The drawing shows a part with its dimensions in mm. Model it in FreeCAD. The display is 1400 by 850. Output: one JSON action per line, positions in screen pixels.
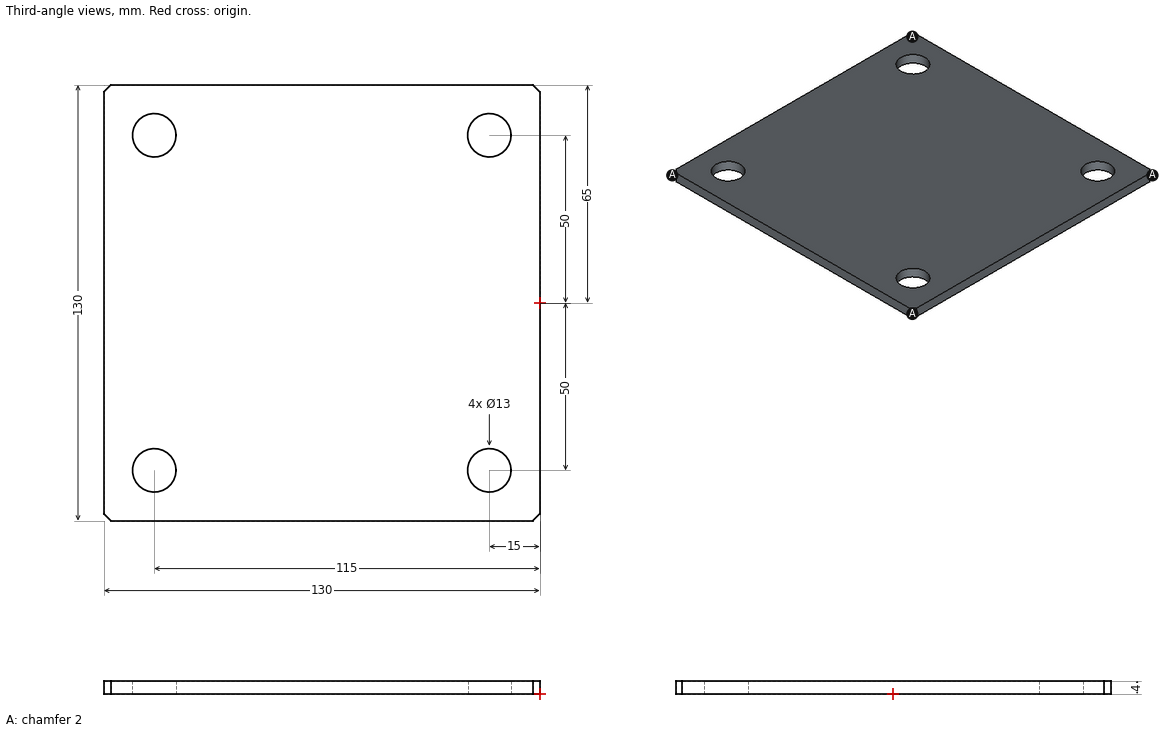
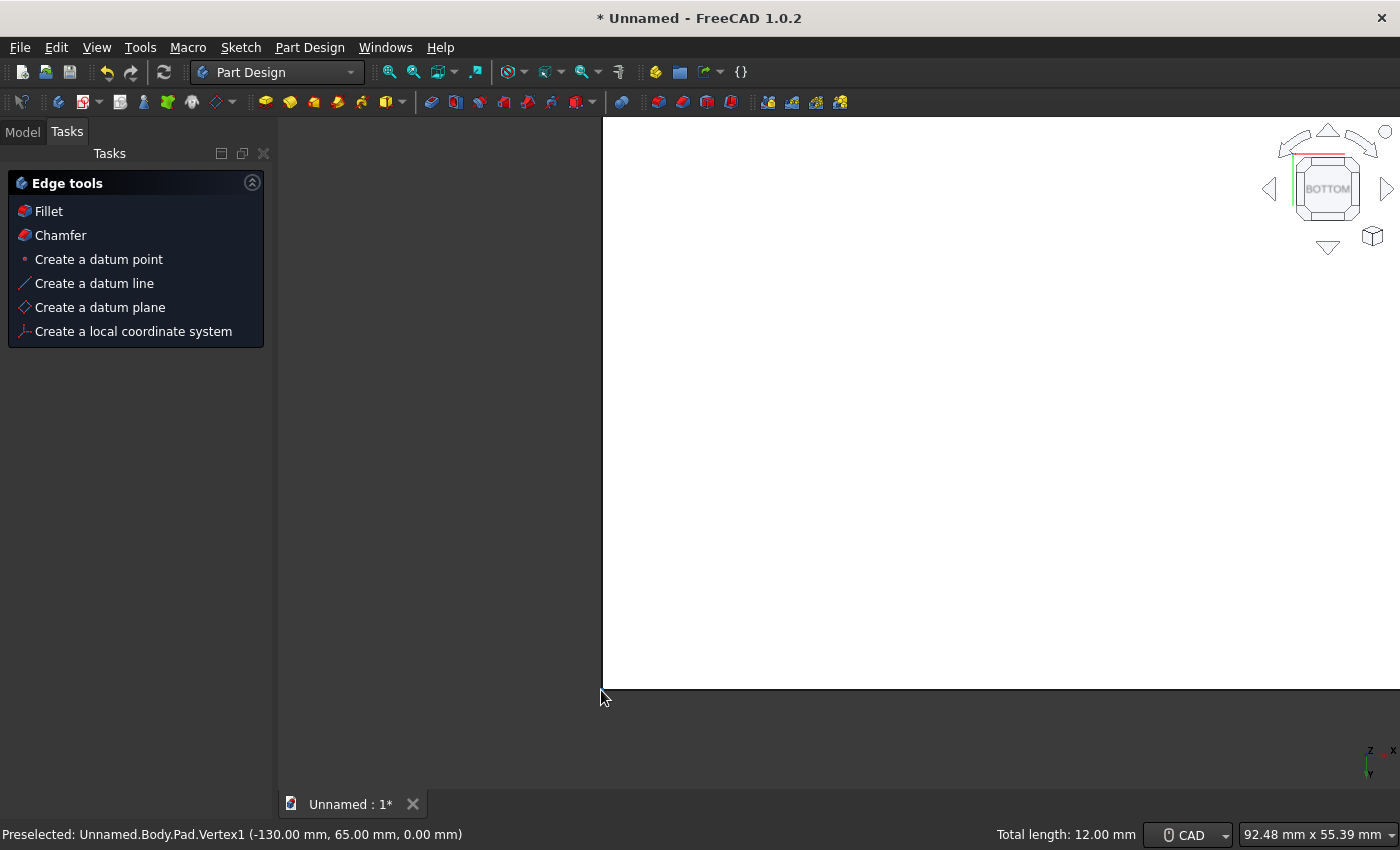
{"action": "left_click", "coordinate": [390, 72]}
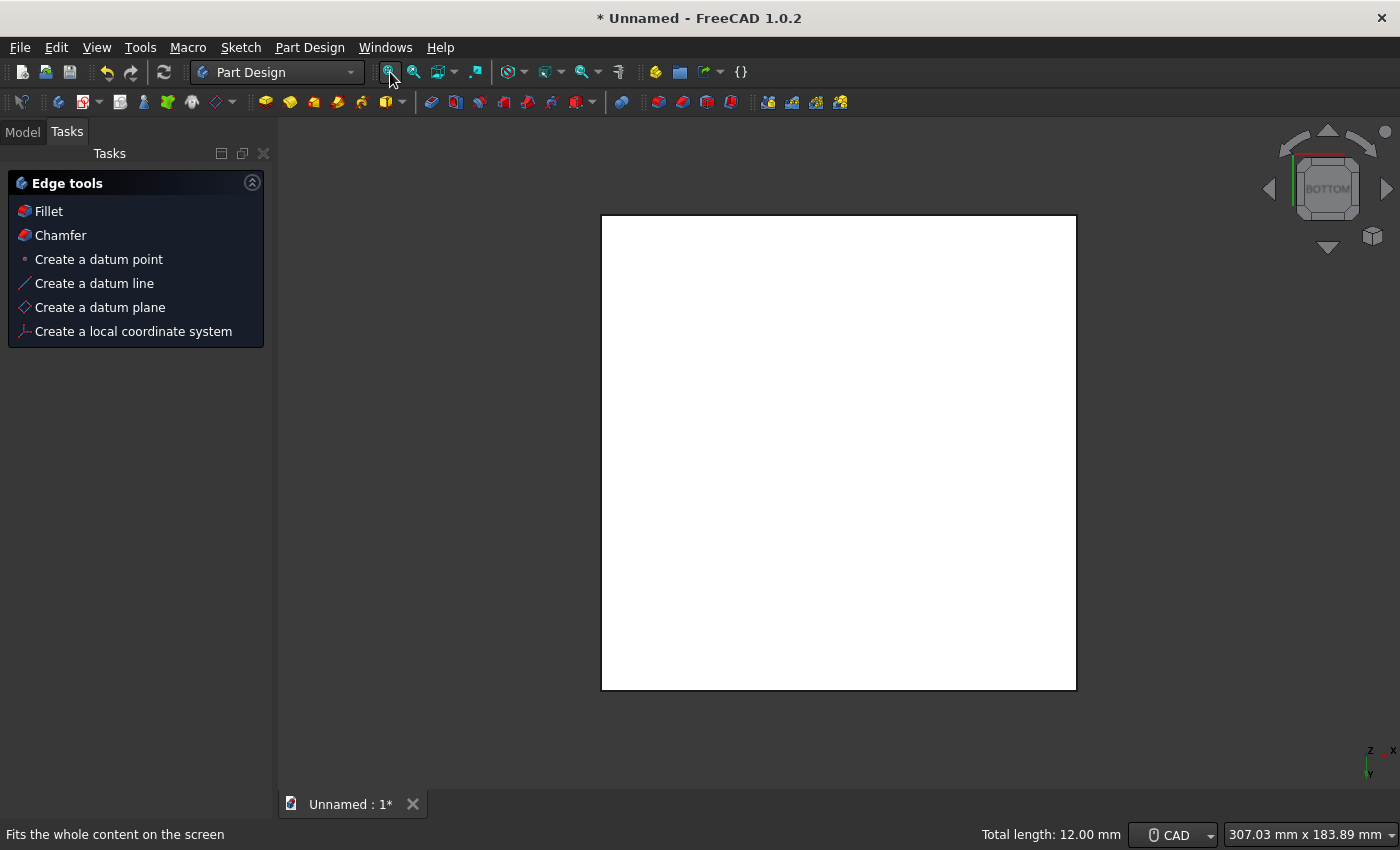
{"action": "key", "text": "4"}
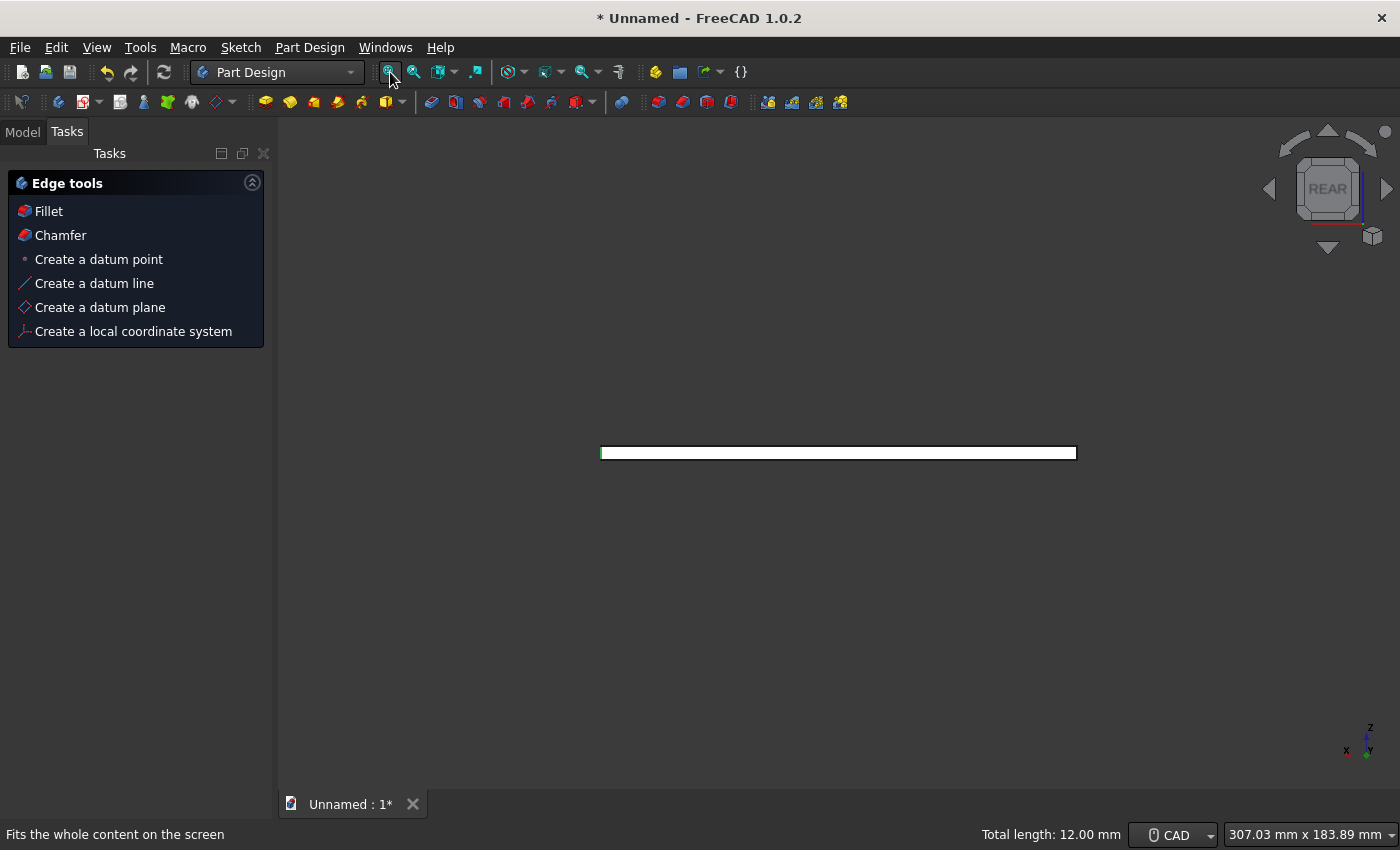
{"action": "left_click", "coordinate": [390, 72]}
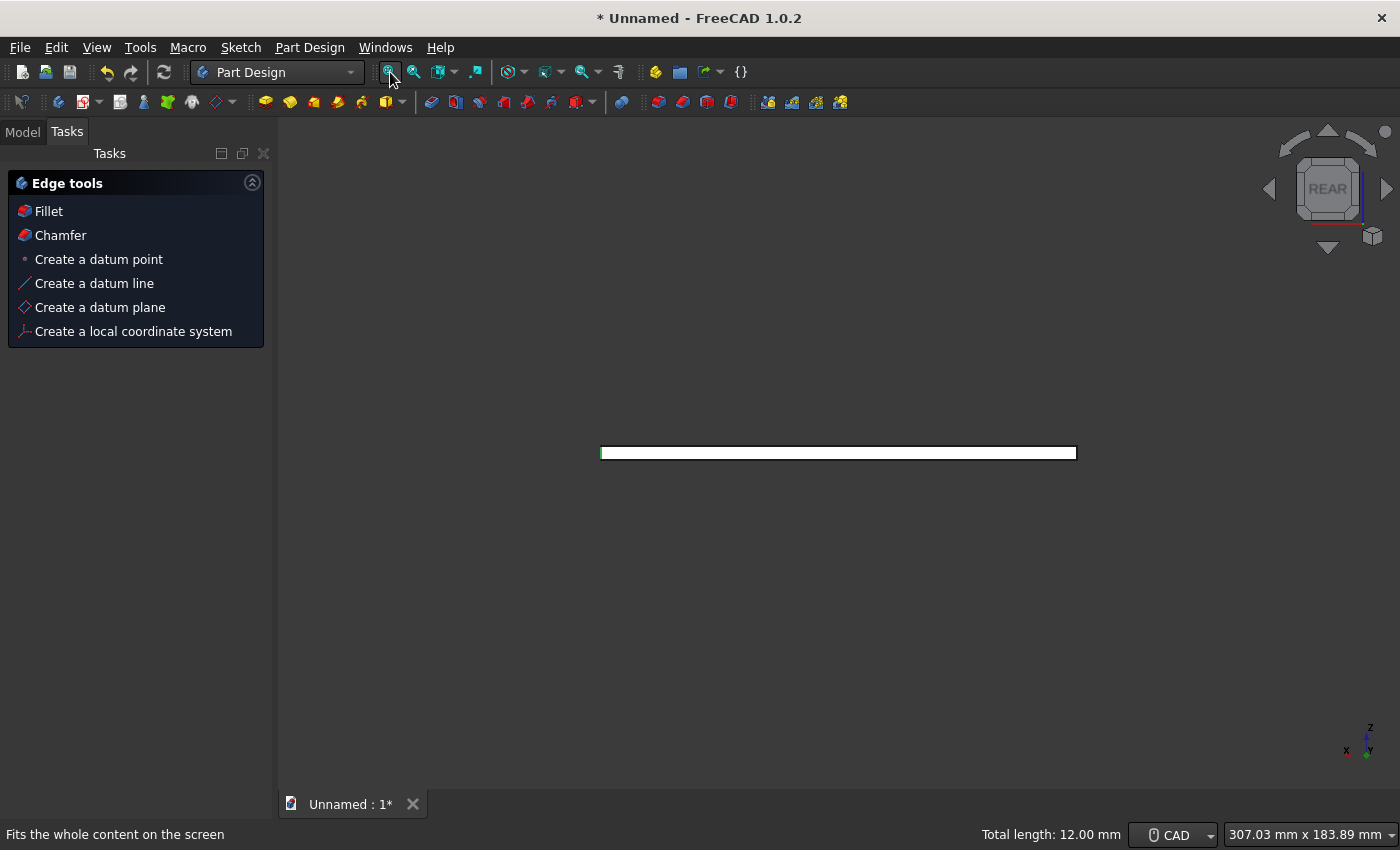
{"action": "left_click", "coordinate": [1077, 452], "text": "ctrl"}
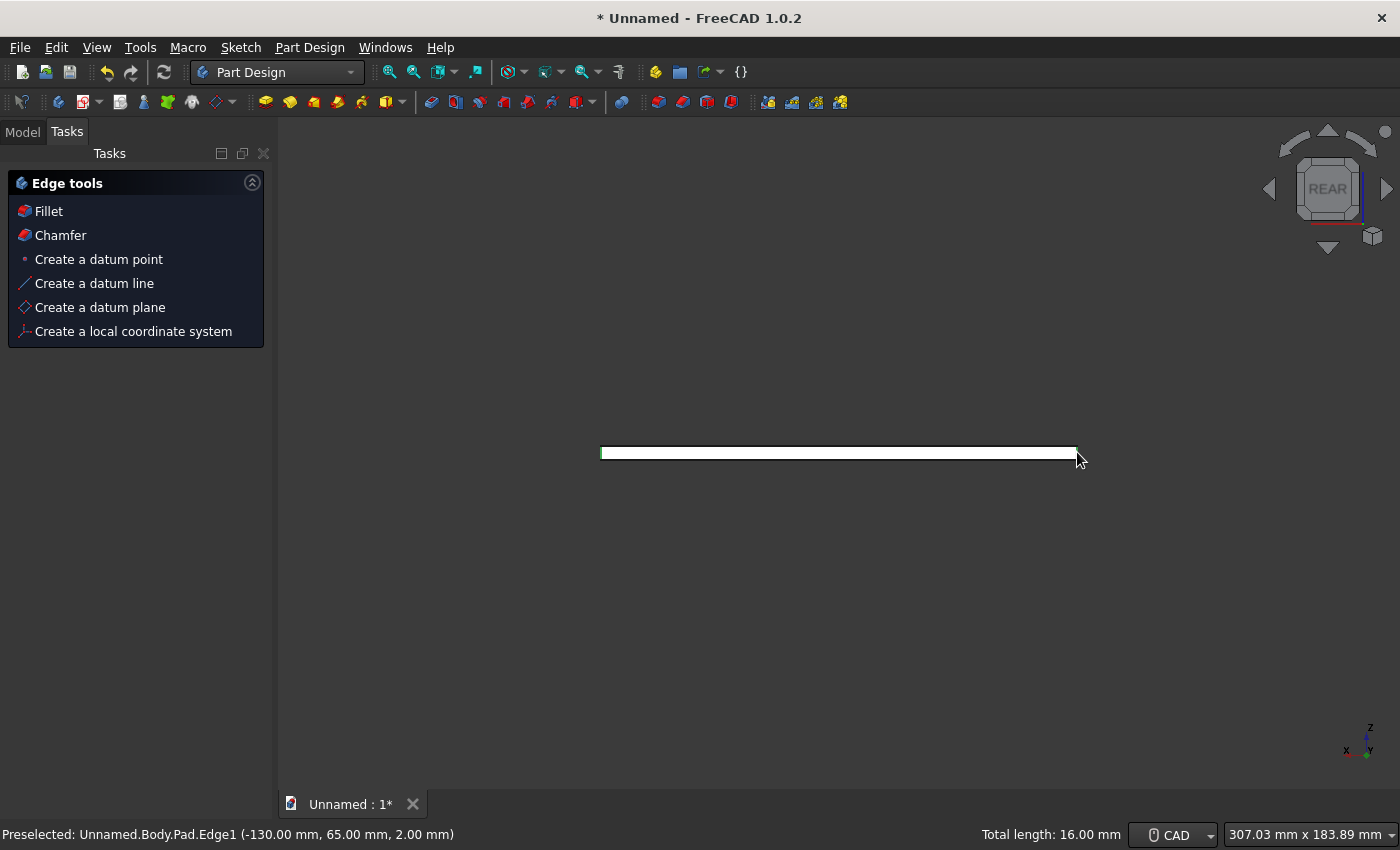
{"action": "left_click", "coordinate": [684, 102]}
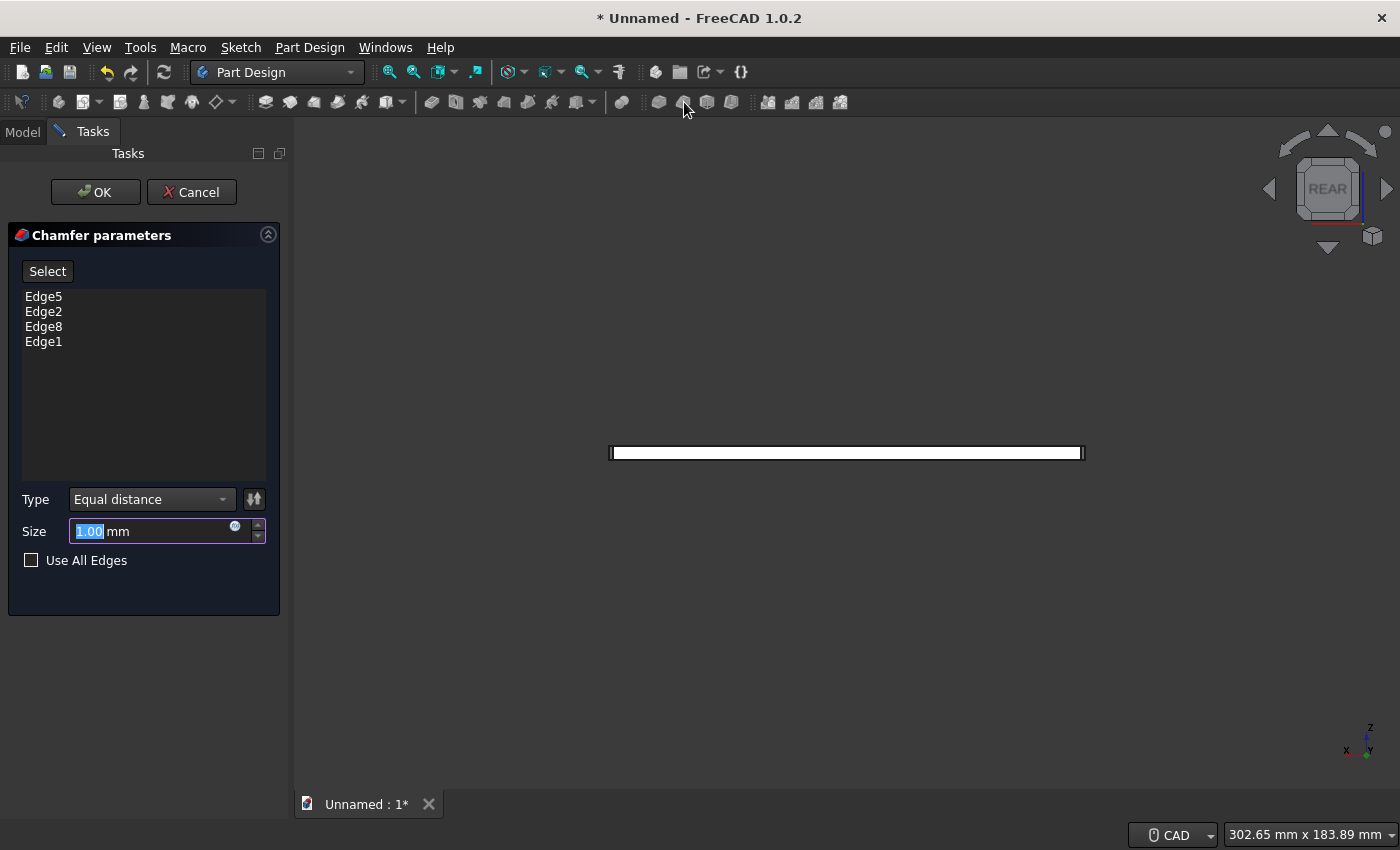
{"action": "type", "text": "2"}
{"action": "key", "text": "Tab"}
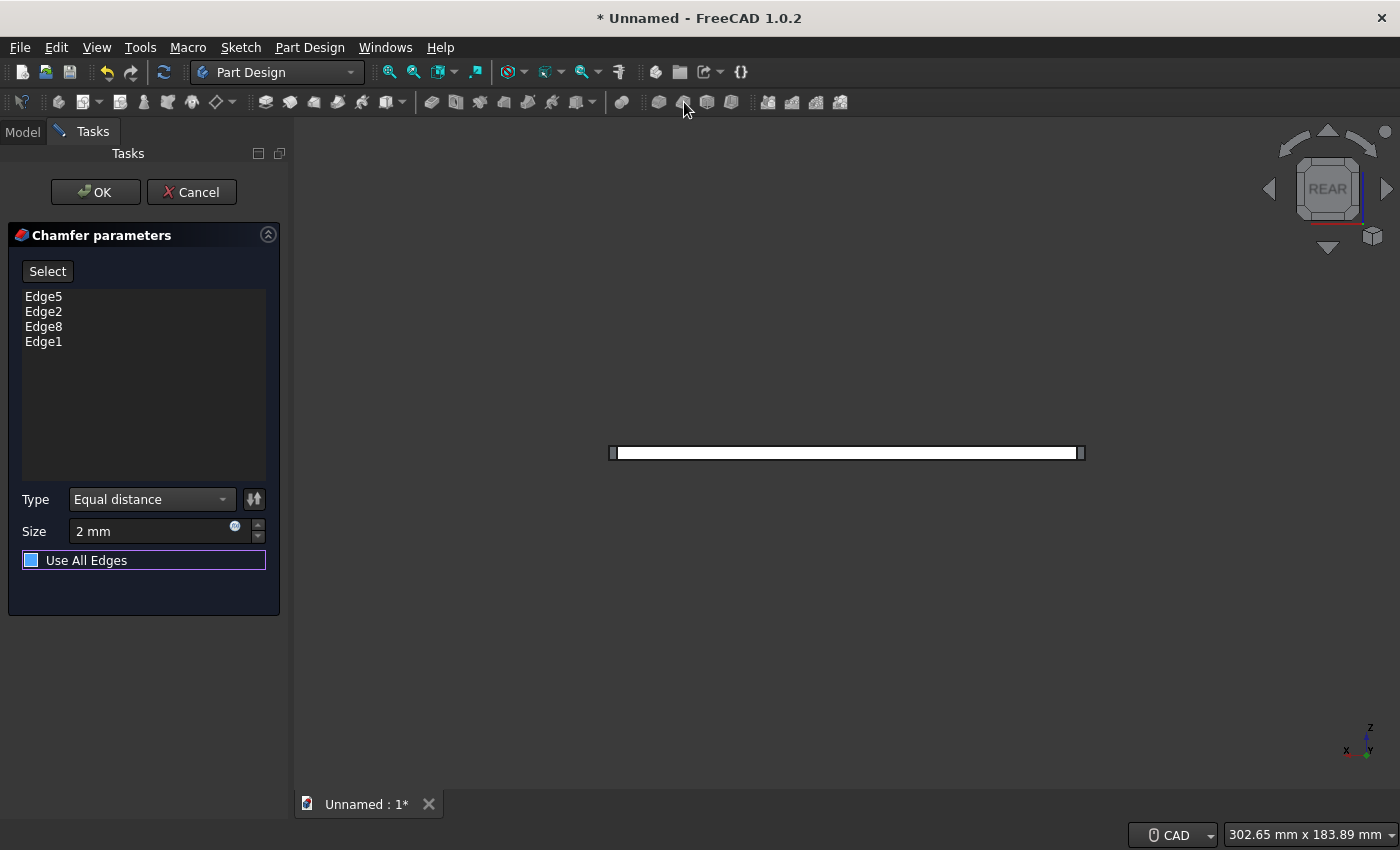
{"action": "left_click", "coordinate": [96, 192]}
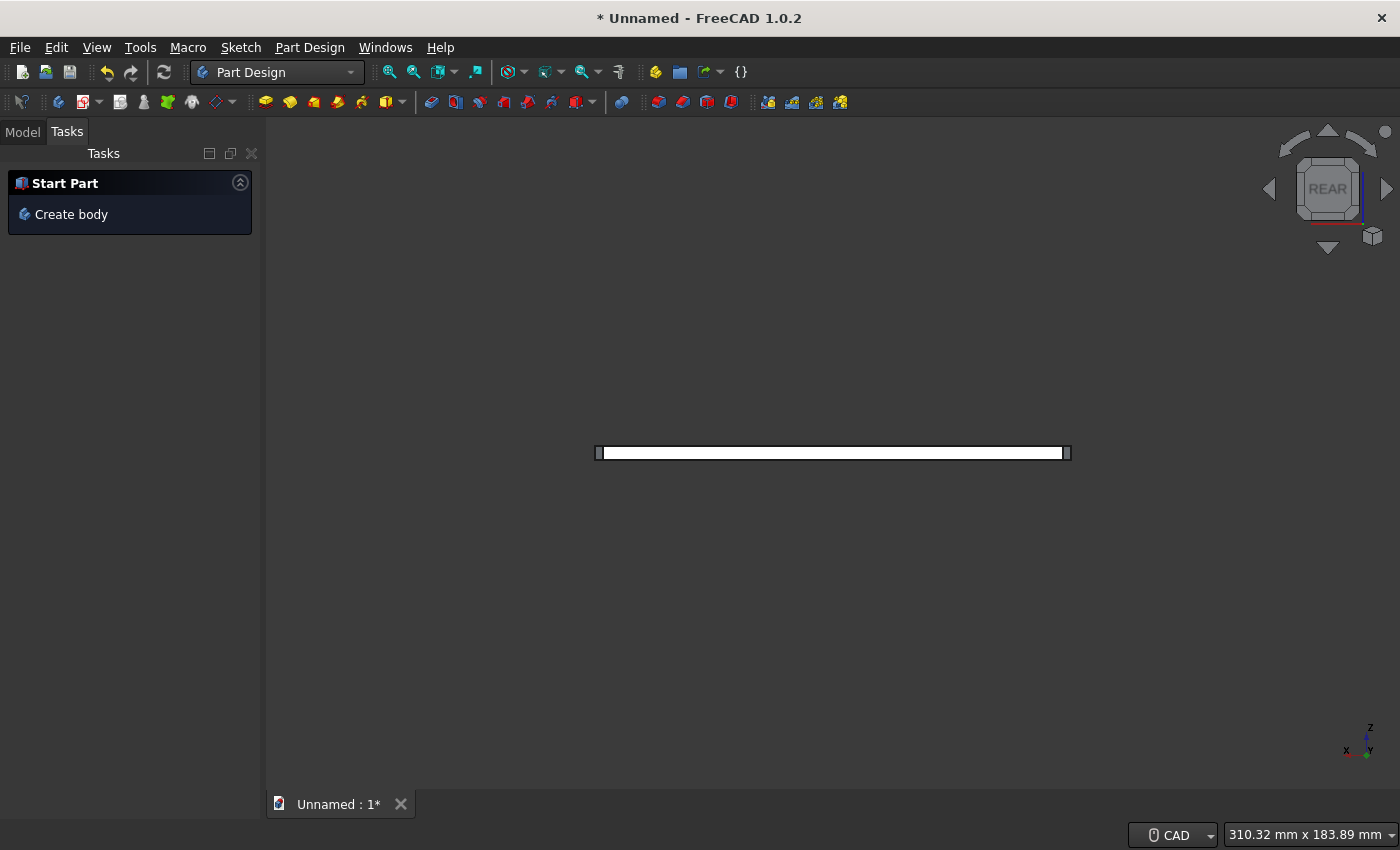
{"action": "left_click", "coordinate": [390, 72]}